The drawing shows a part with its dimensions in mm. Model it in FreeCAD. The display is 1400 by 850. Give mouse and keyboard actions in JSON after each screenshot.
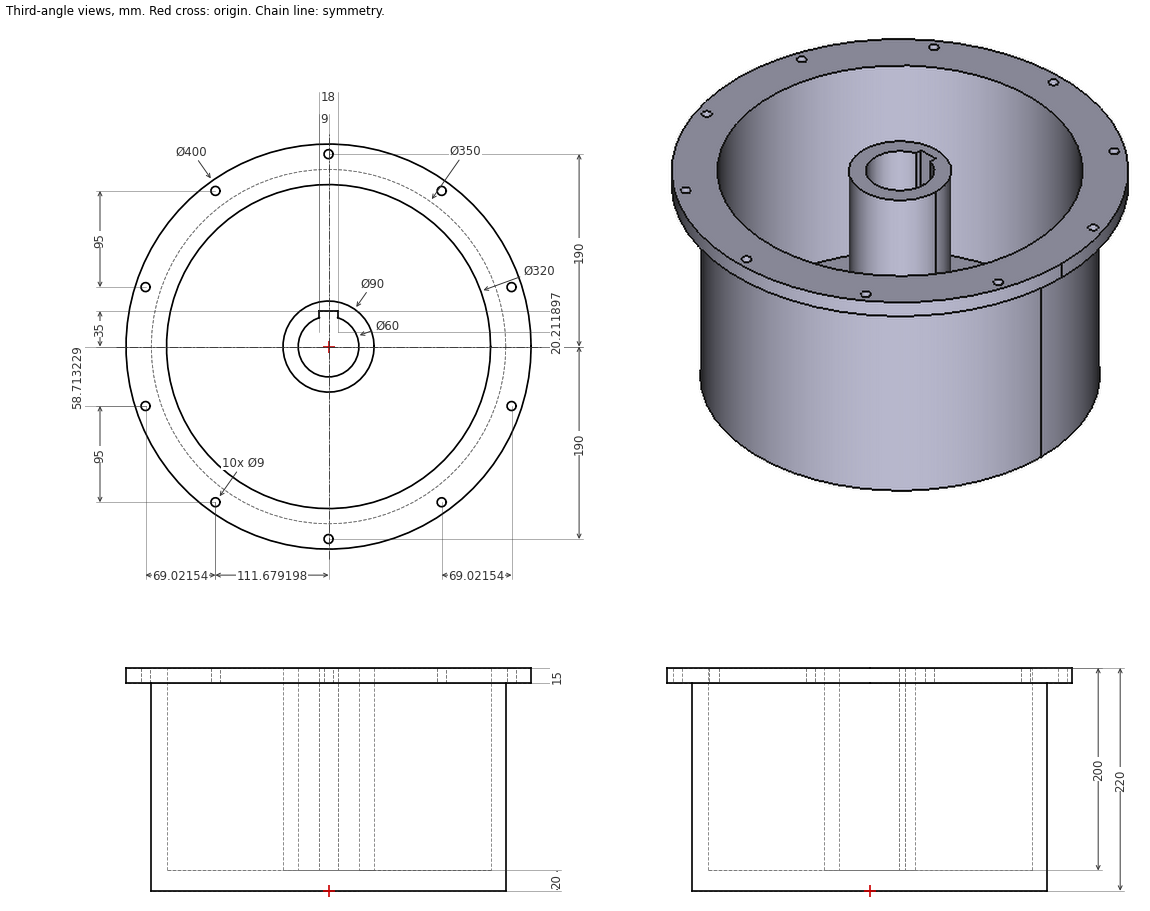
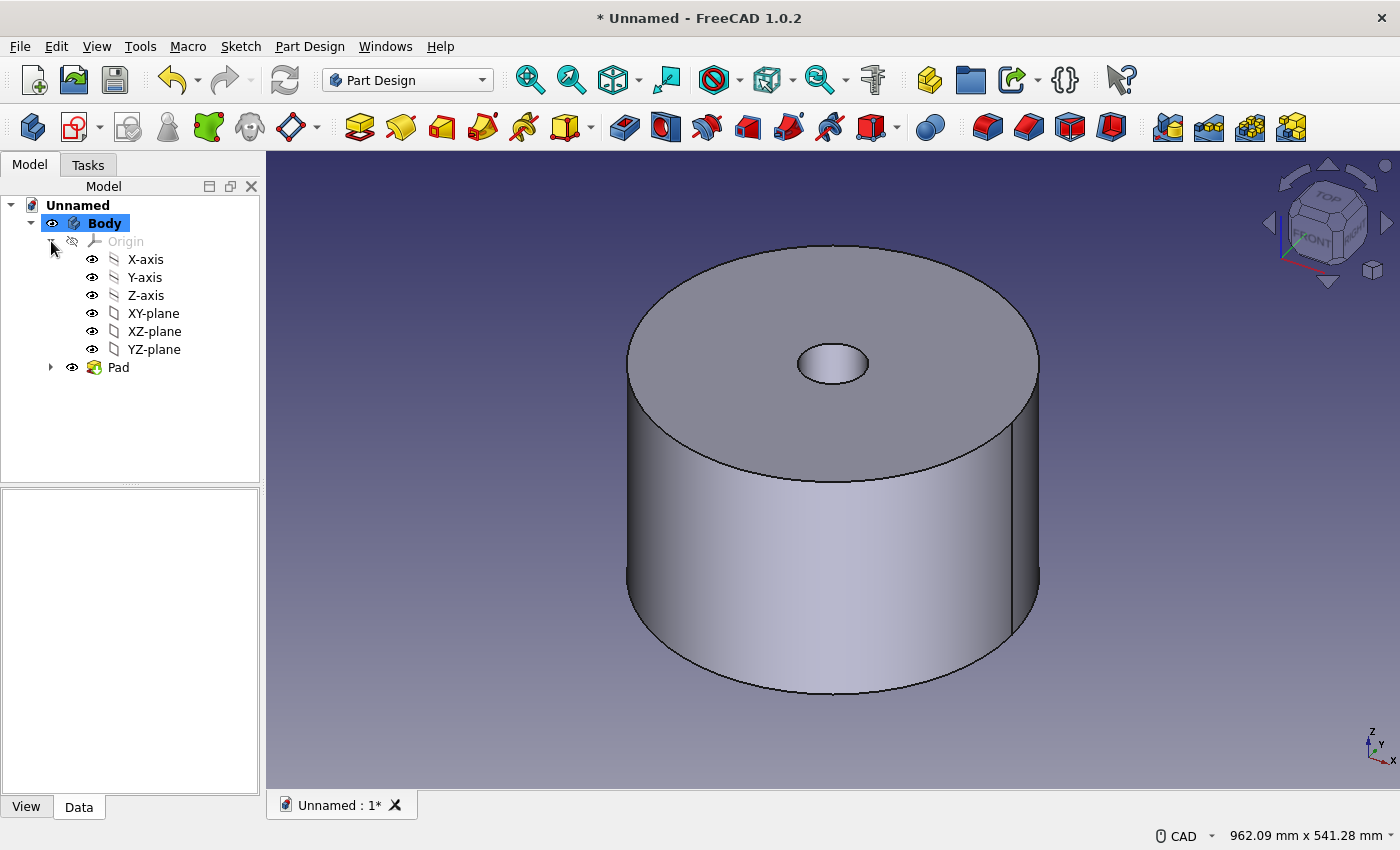
{"action": "left_click", "coordinate": [137, 313]}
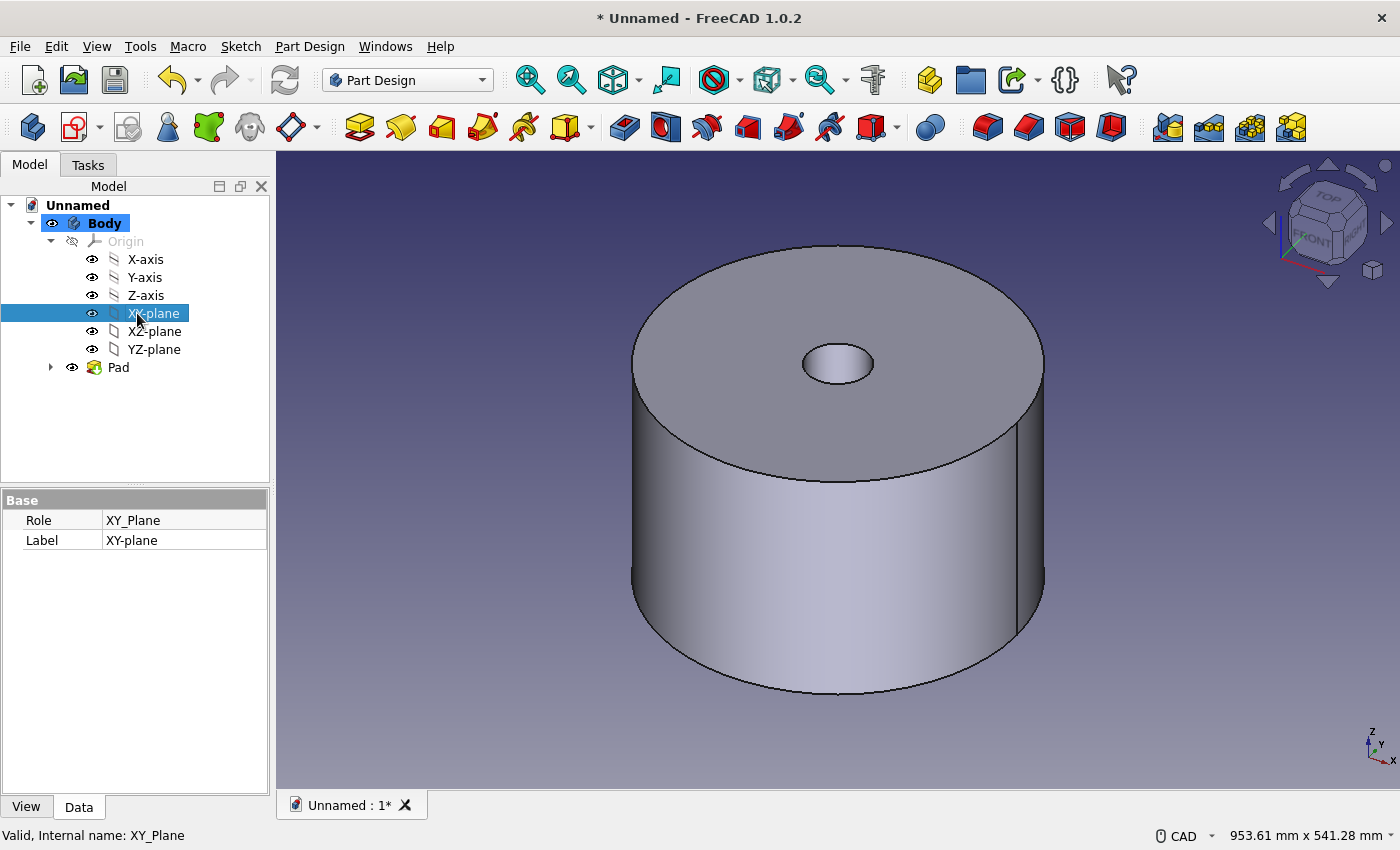
{"action": "left_click", "coordinate": [290, 128]}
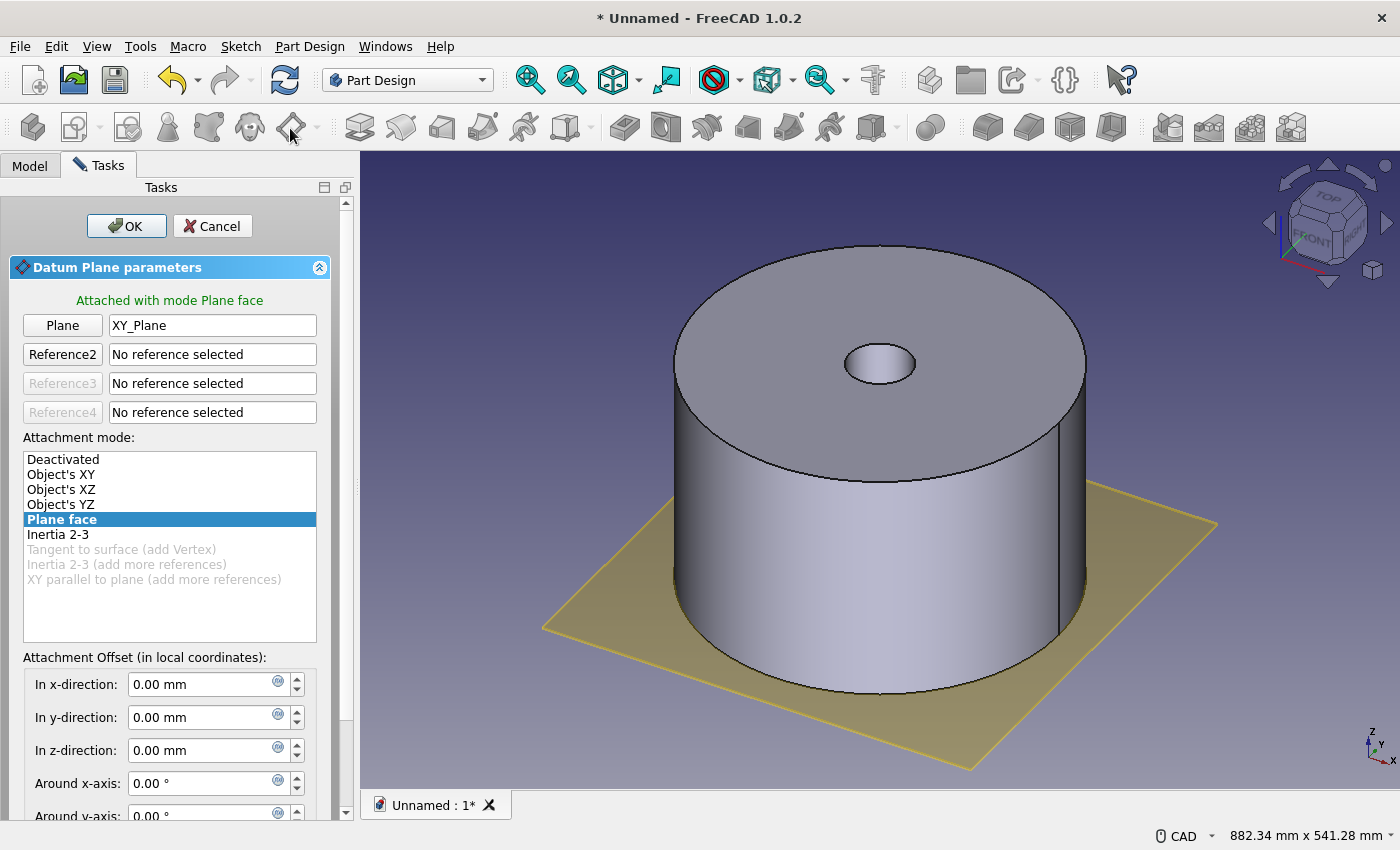
{"action": "triple_click", "coordinate": [210, 750]}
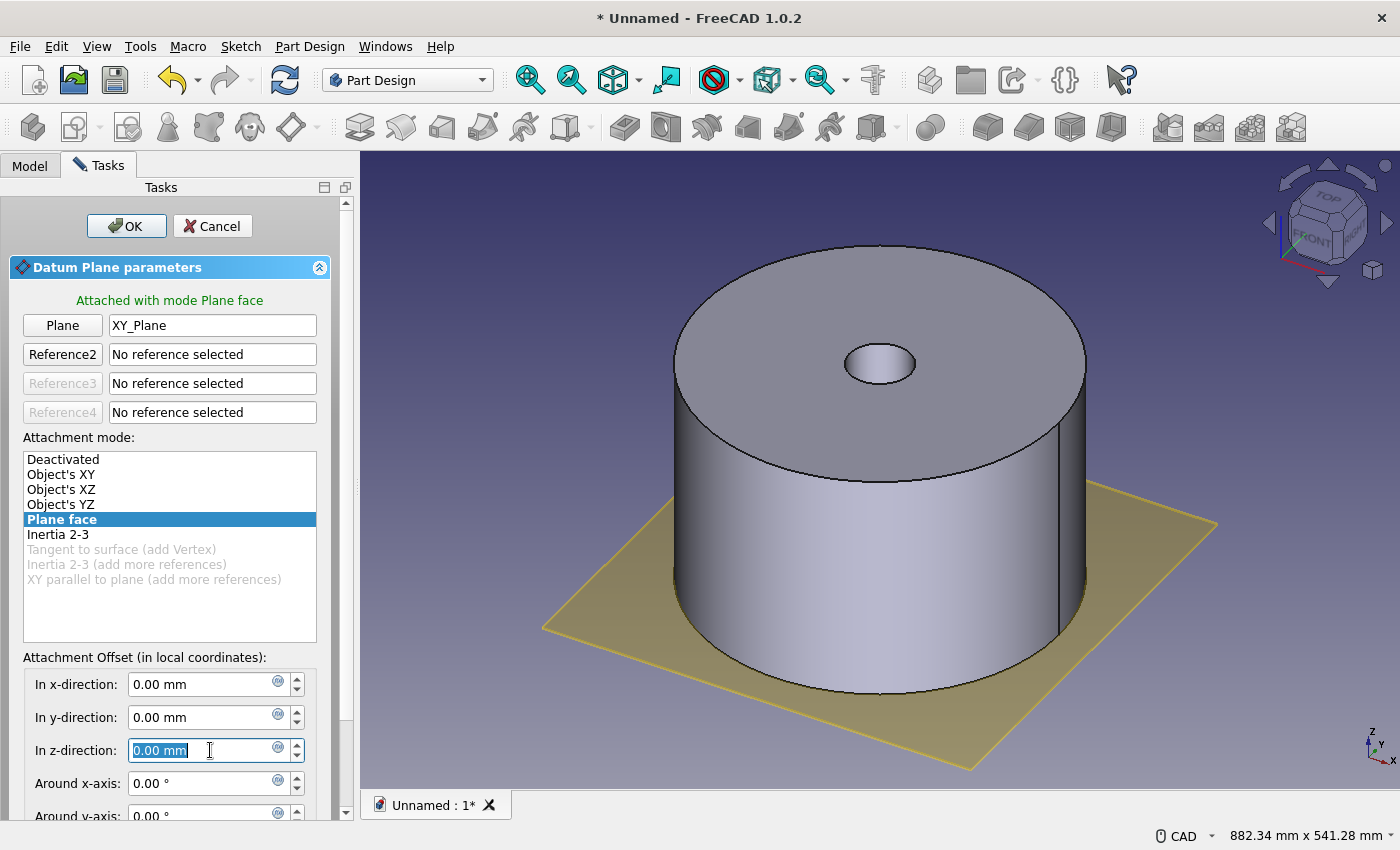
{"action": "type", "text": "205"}
{"action": "key", "text": "Tab"}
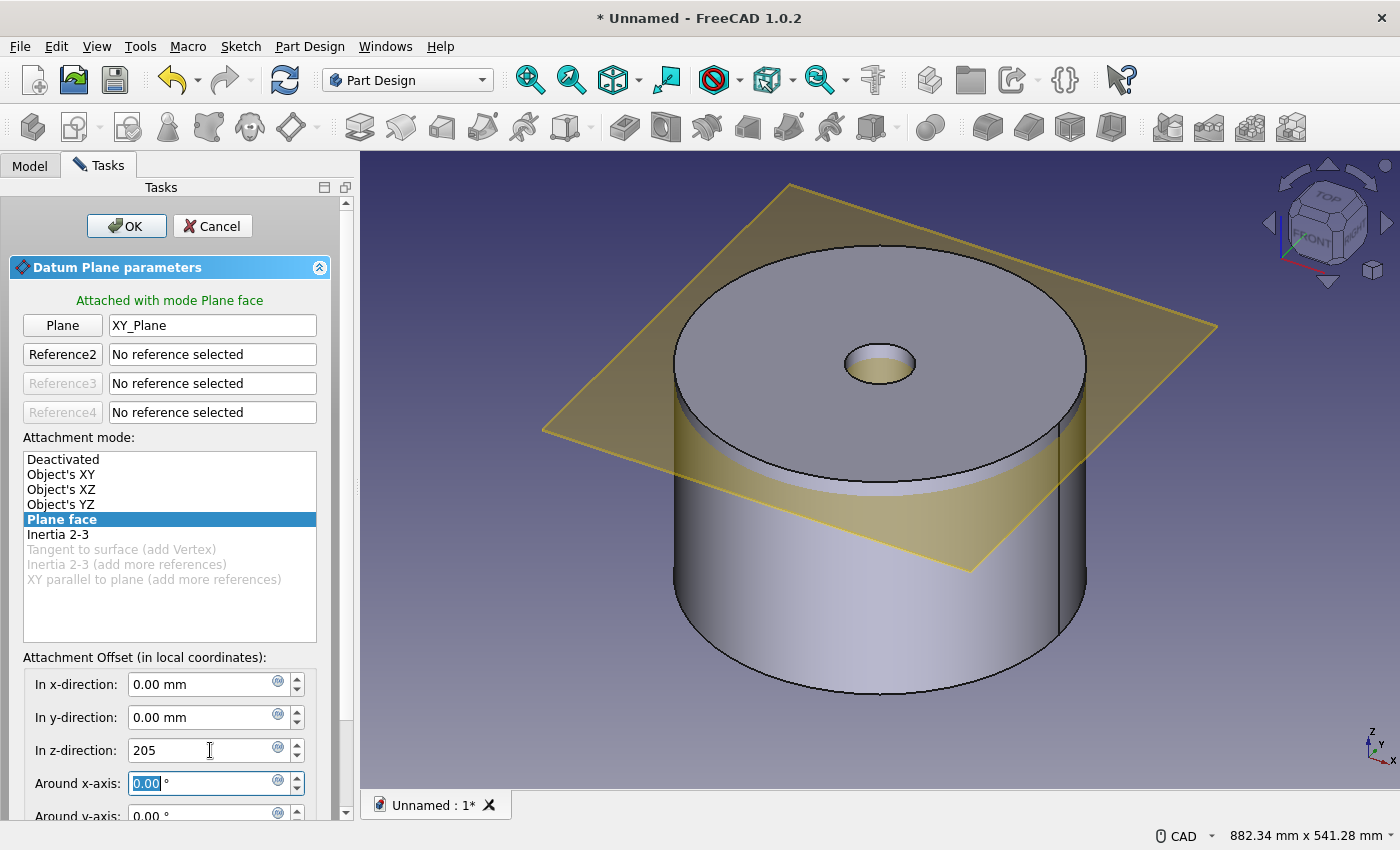
{"action": "left_click", "coordinate": [127, 226]}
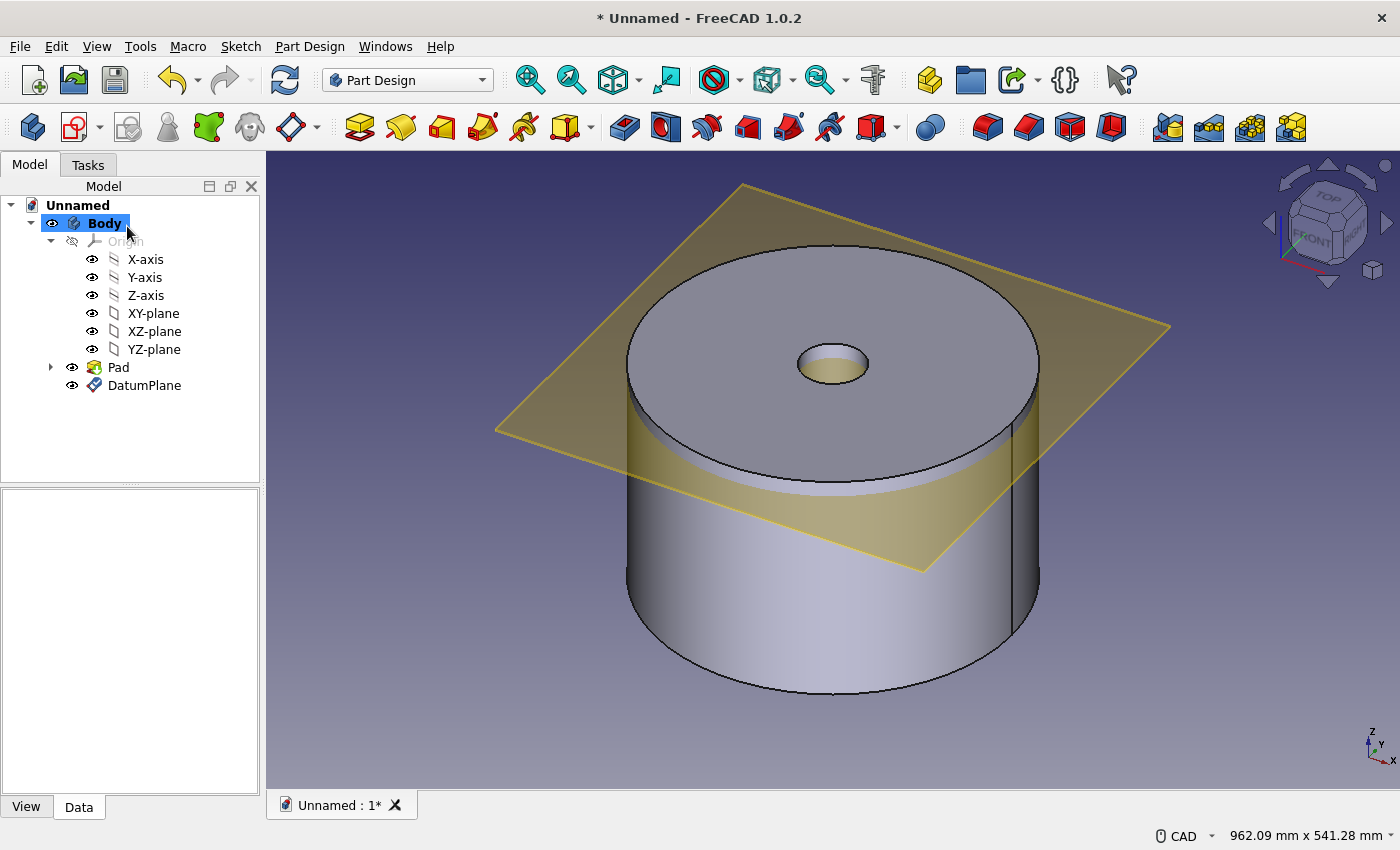
{"action": "left_click", "coordinate": [117, 385]}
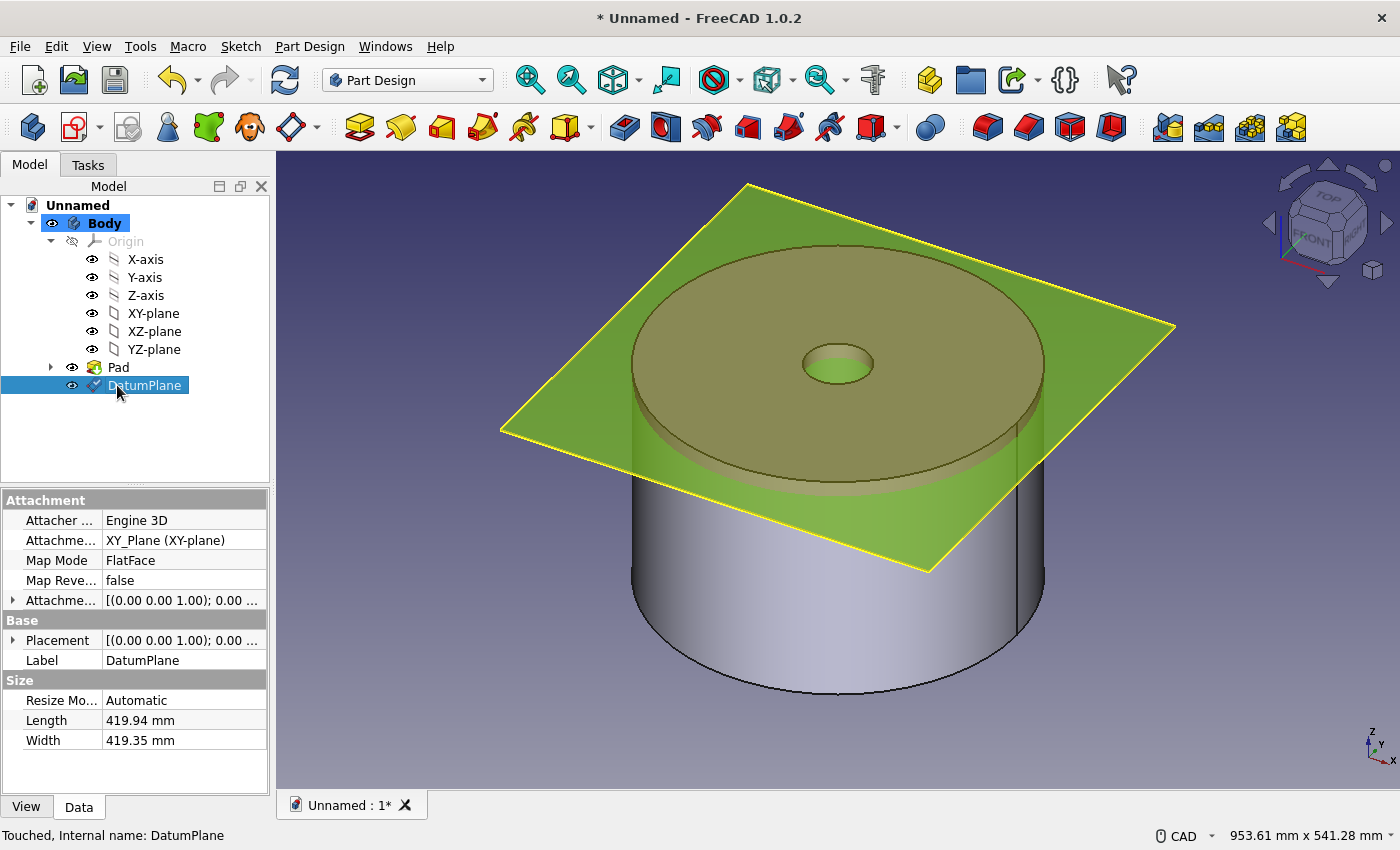
{"action": "left_click", "coordinate": [74, 128]}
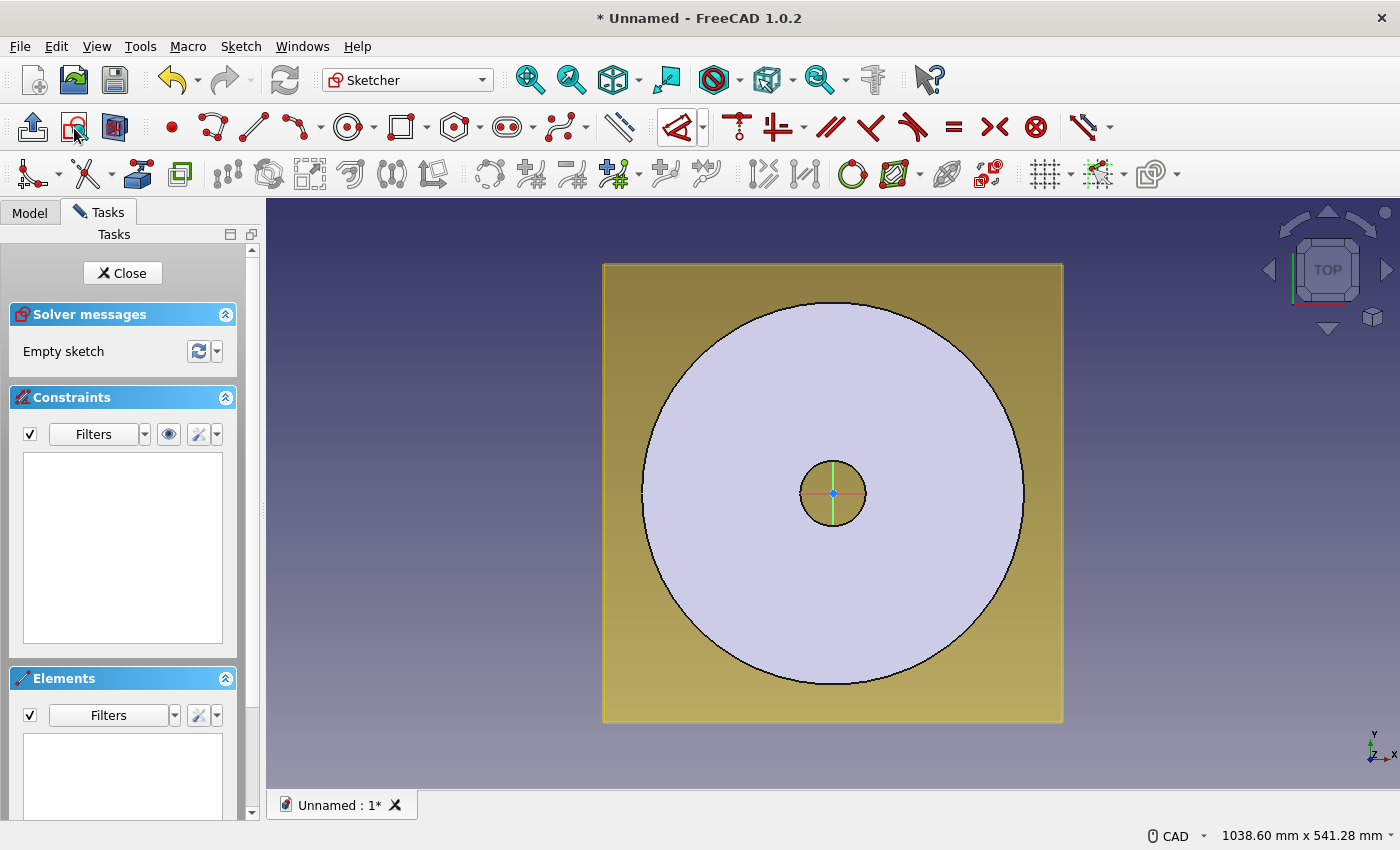
{"action": "left_click", "coordinate": [115, 128]}